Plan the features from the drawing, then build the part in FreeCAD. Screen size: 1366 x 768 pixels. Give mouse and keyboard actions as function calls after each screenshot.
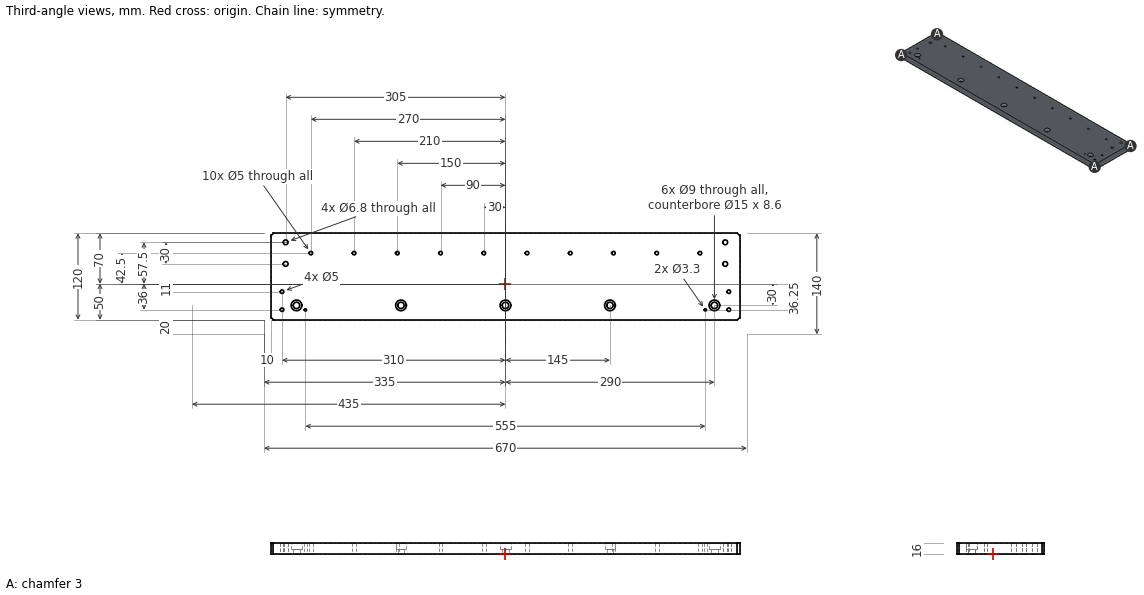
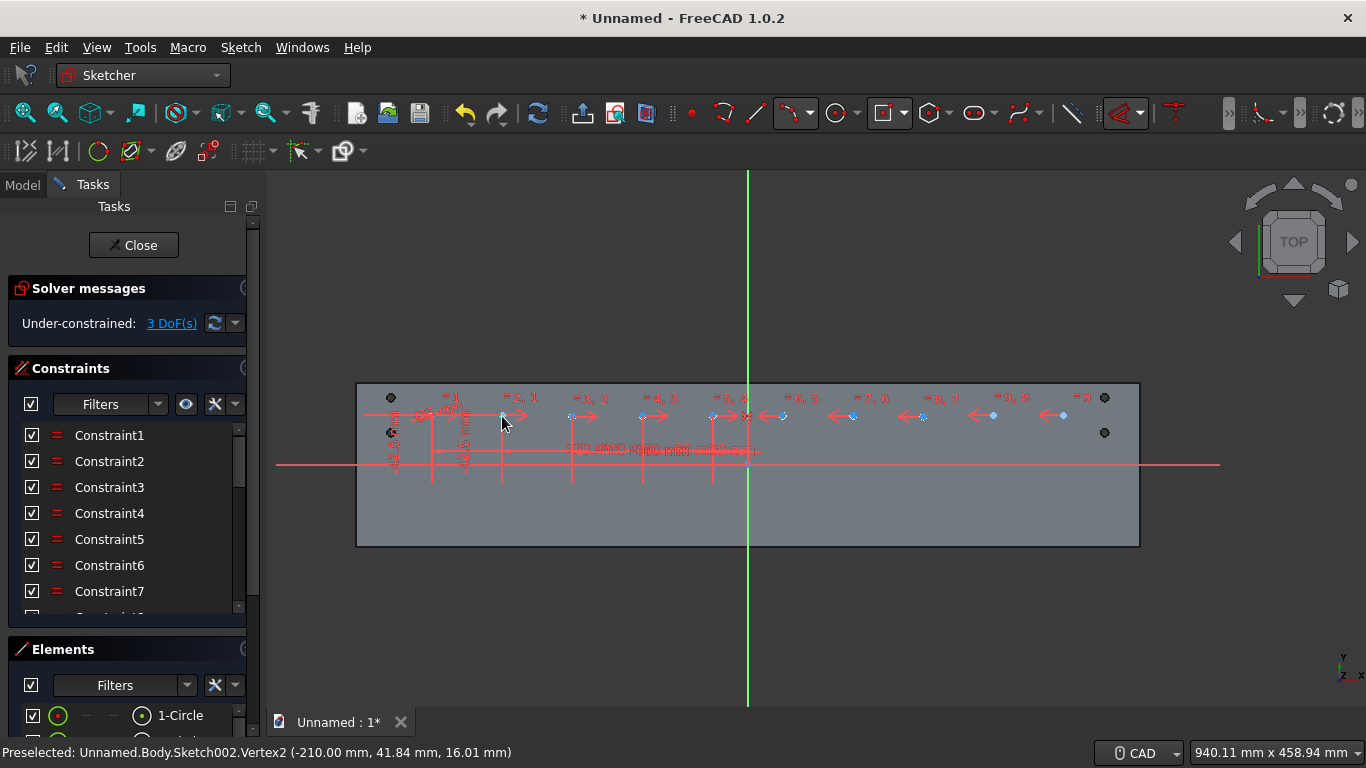
click(572, 417)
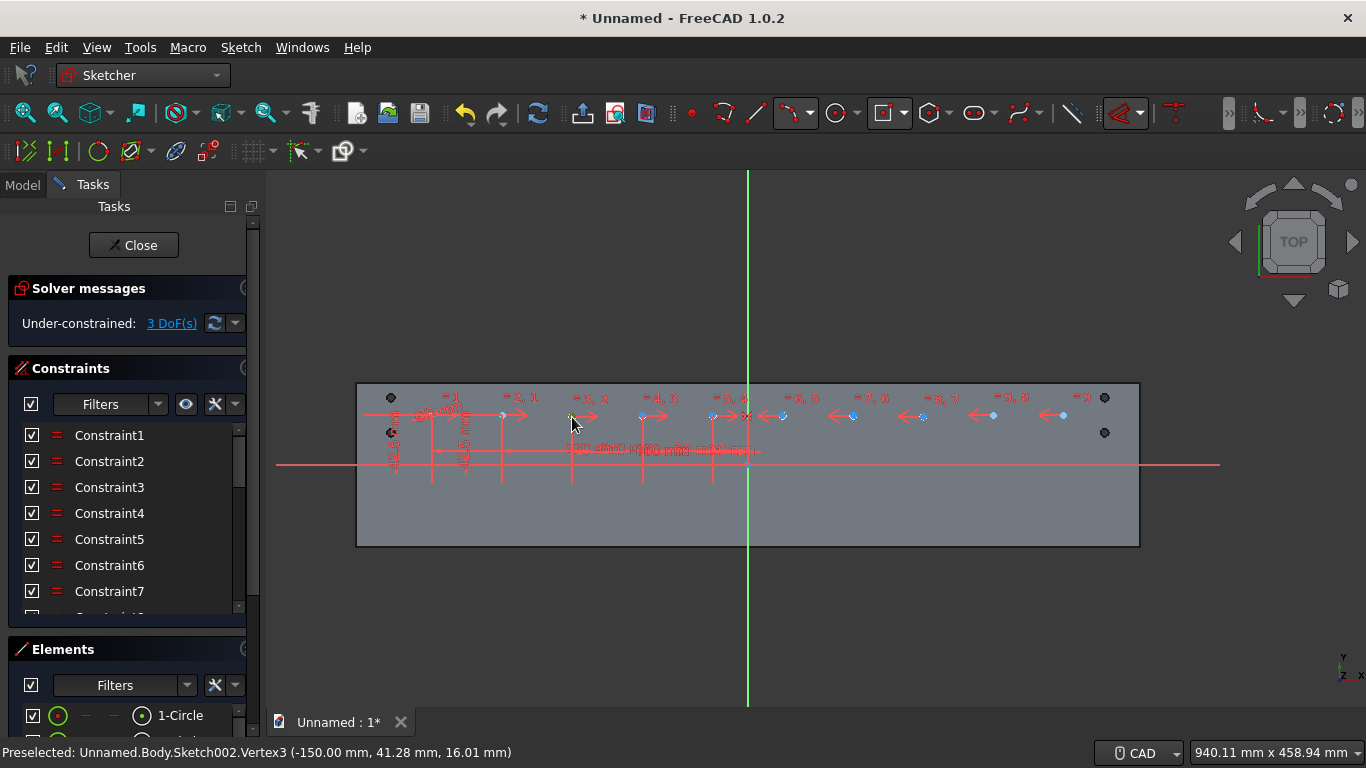
click(1142, 114)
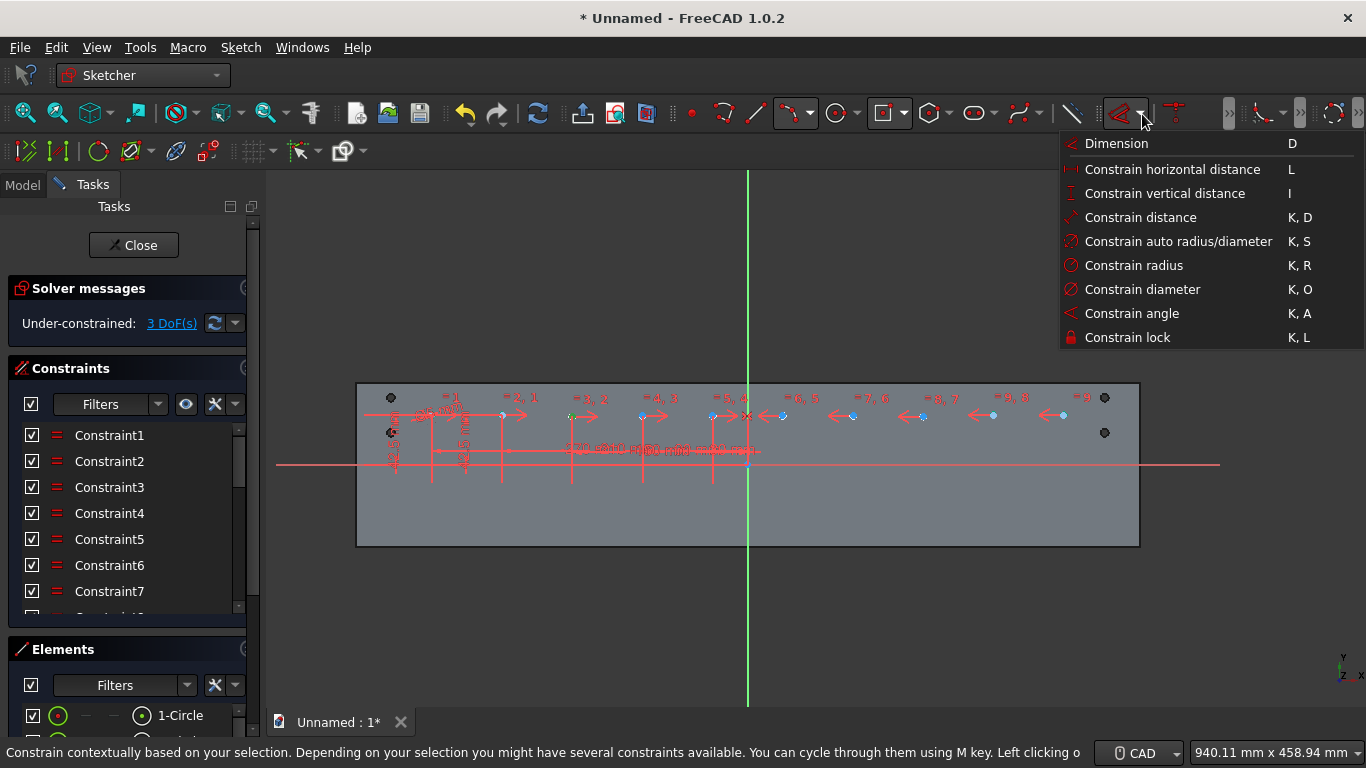
click(1212, 193)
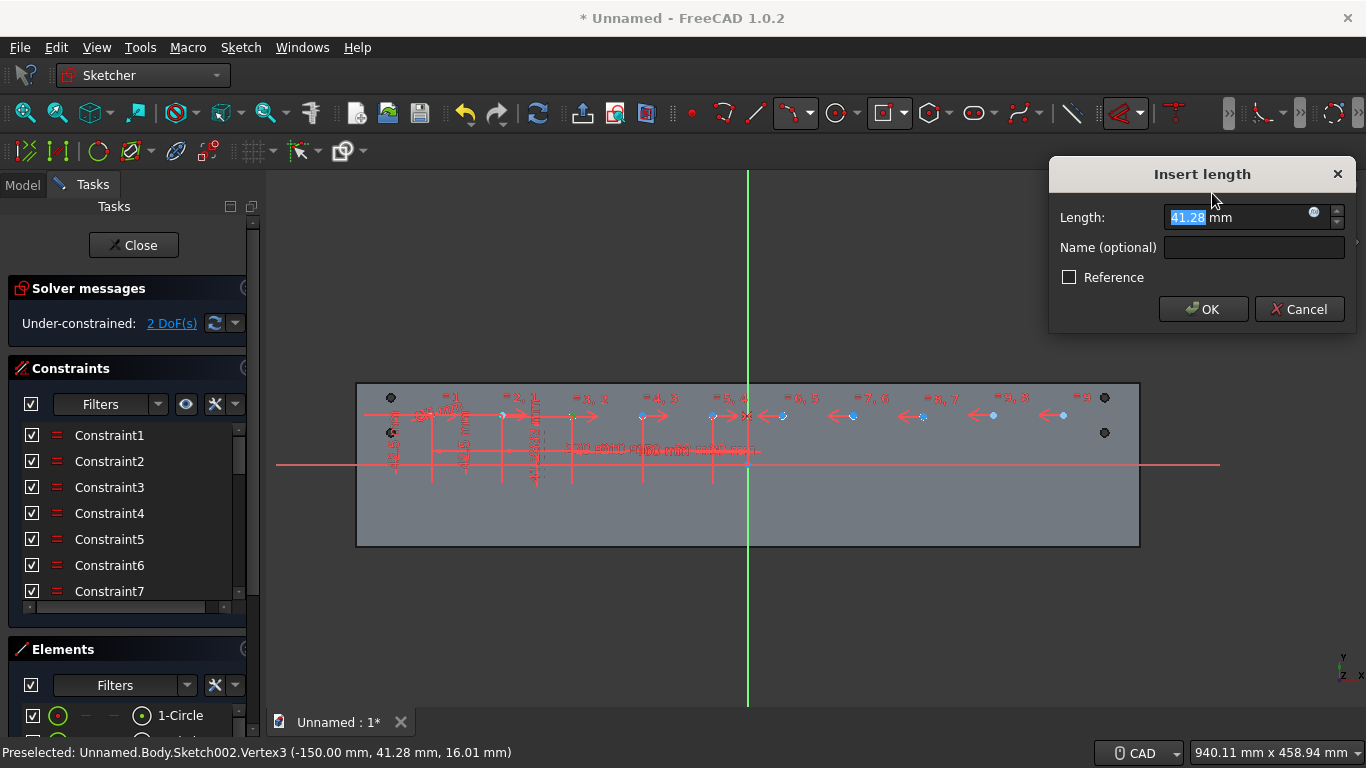
text(42.5)
key(Return)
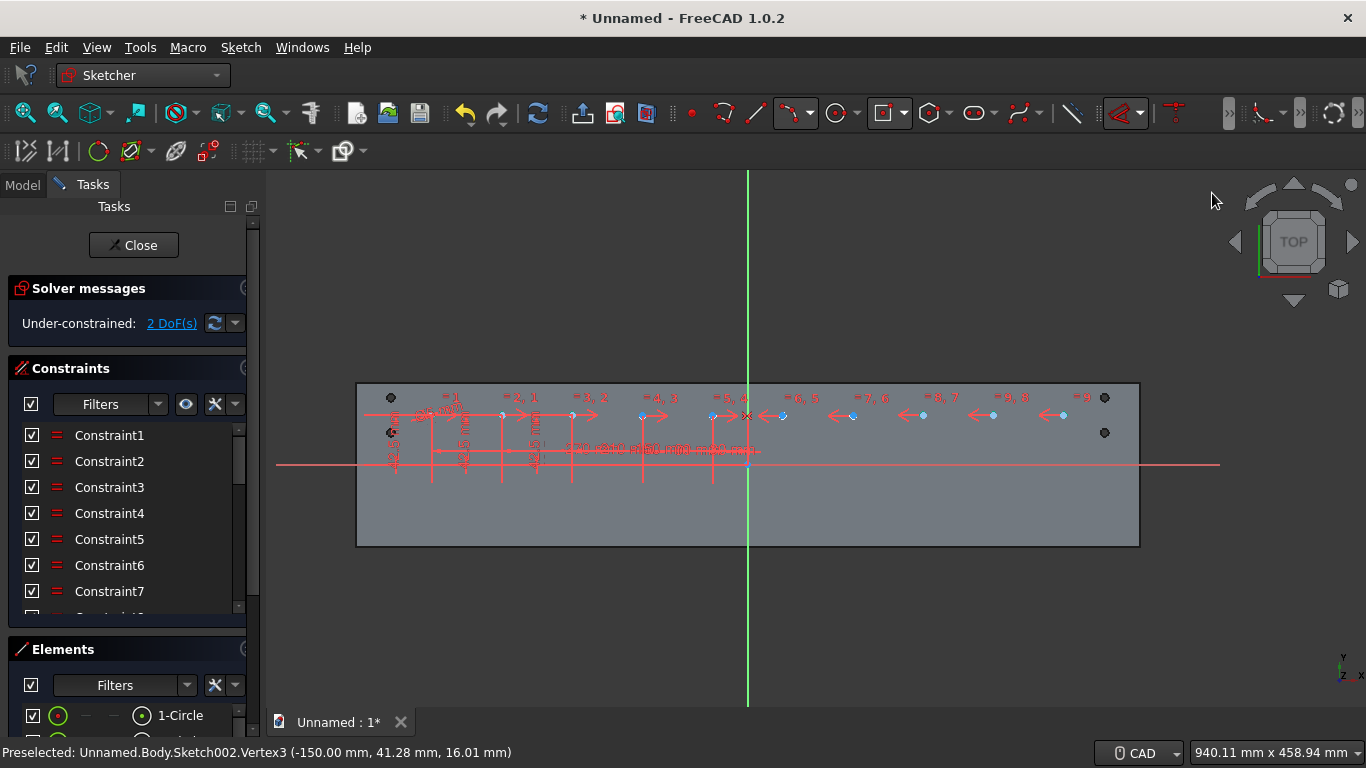
click(643, 416)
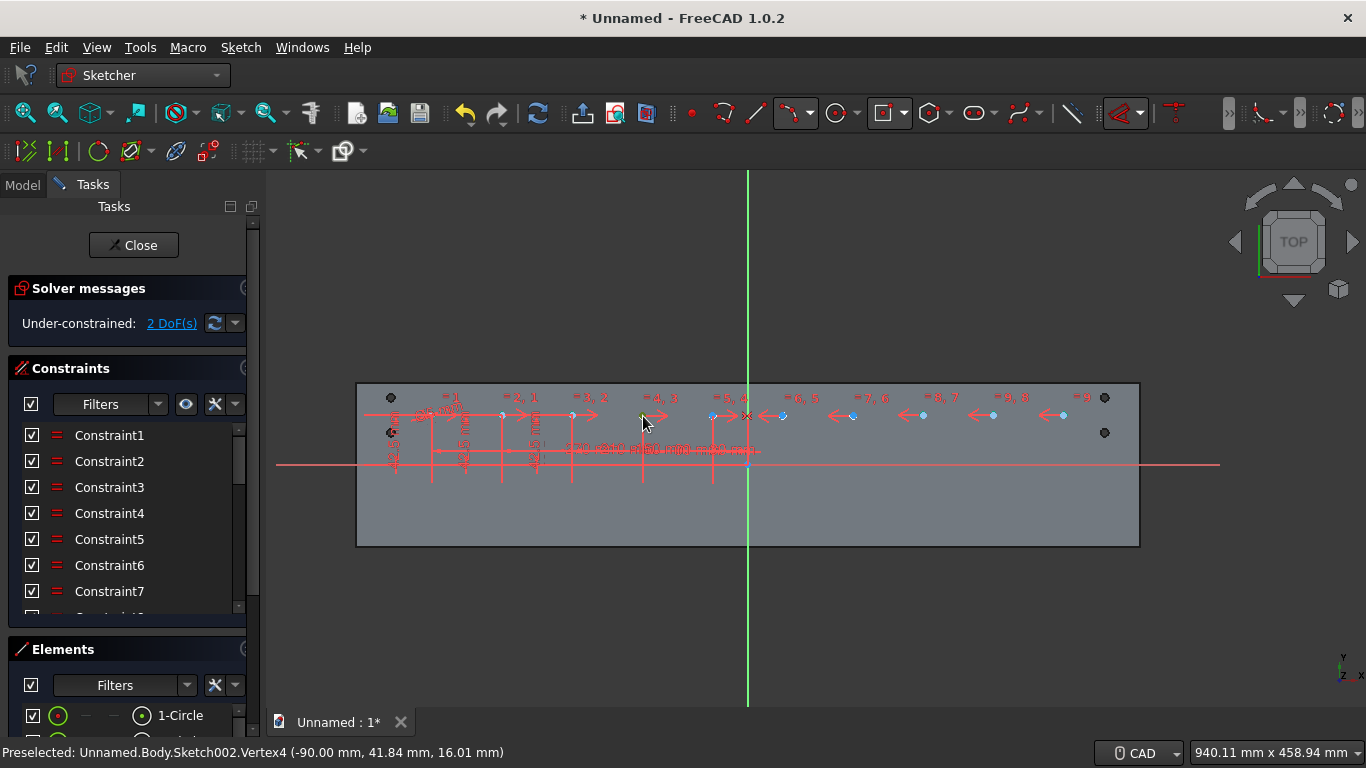
key(i)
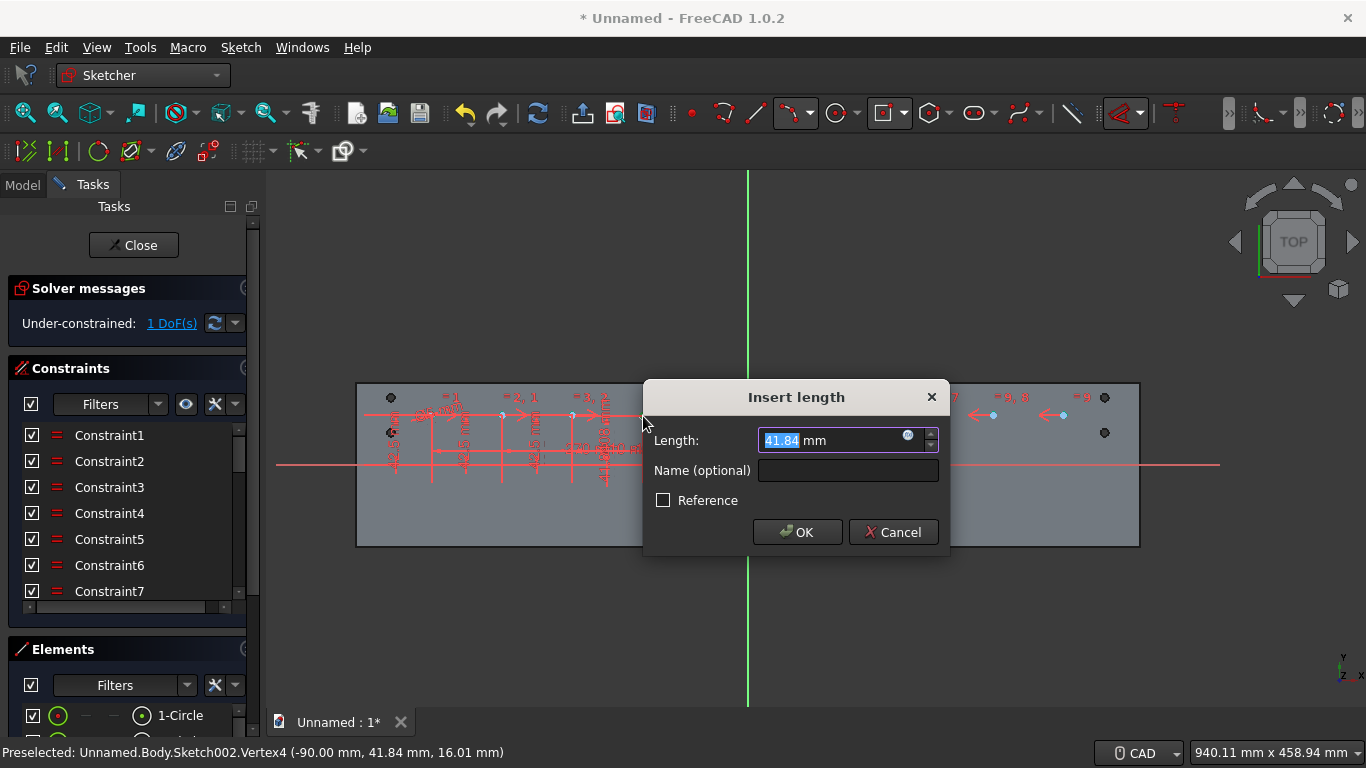
text(42.5)
key(Return)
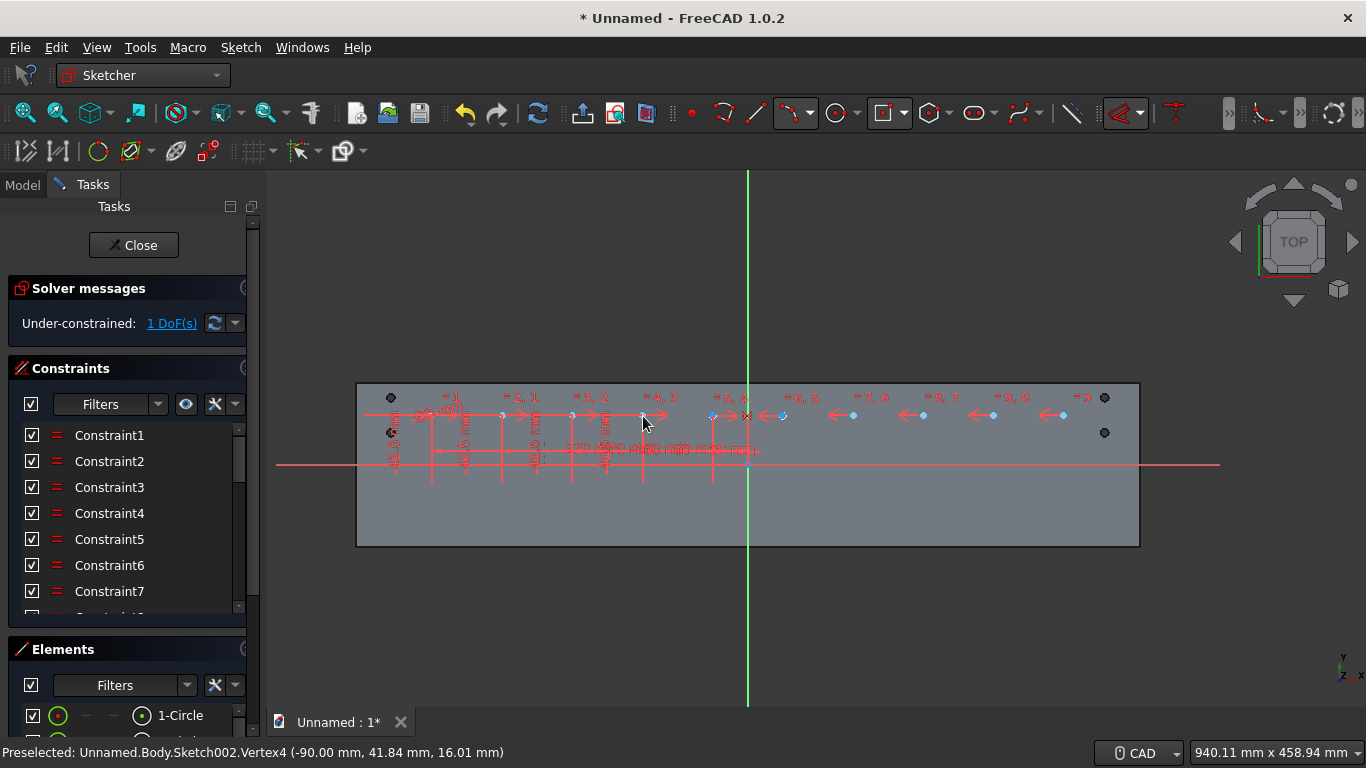
click(713, 416)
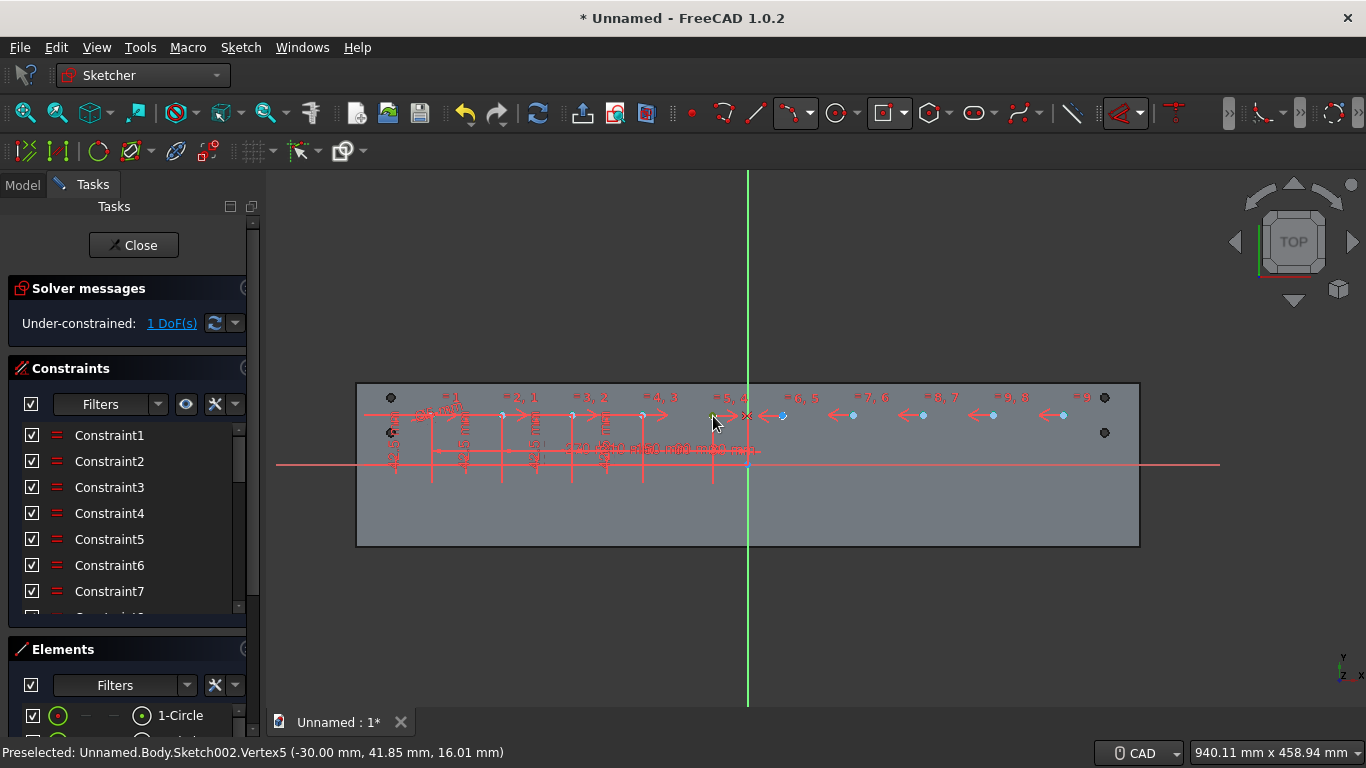
key(i)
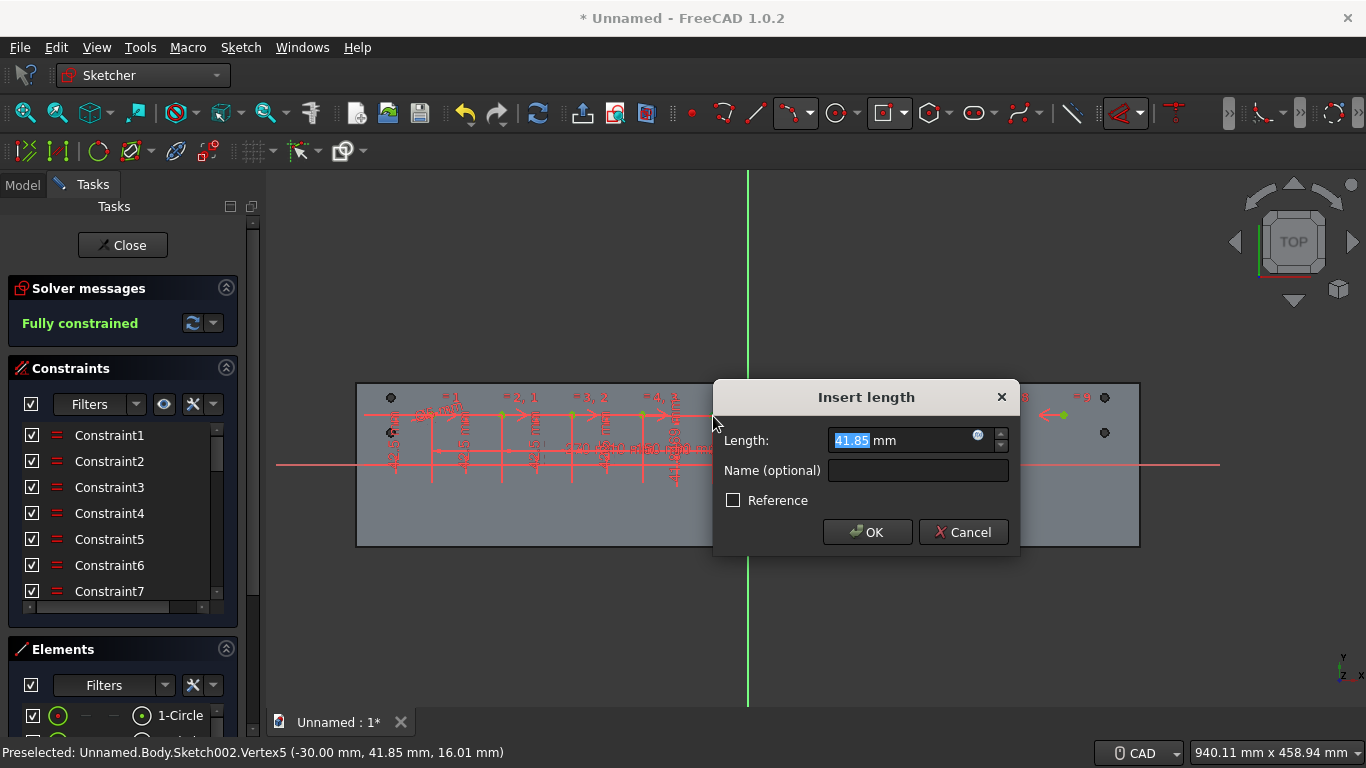
text(42.5)
key(Return)